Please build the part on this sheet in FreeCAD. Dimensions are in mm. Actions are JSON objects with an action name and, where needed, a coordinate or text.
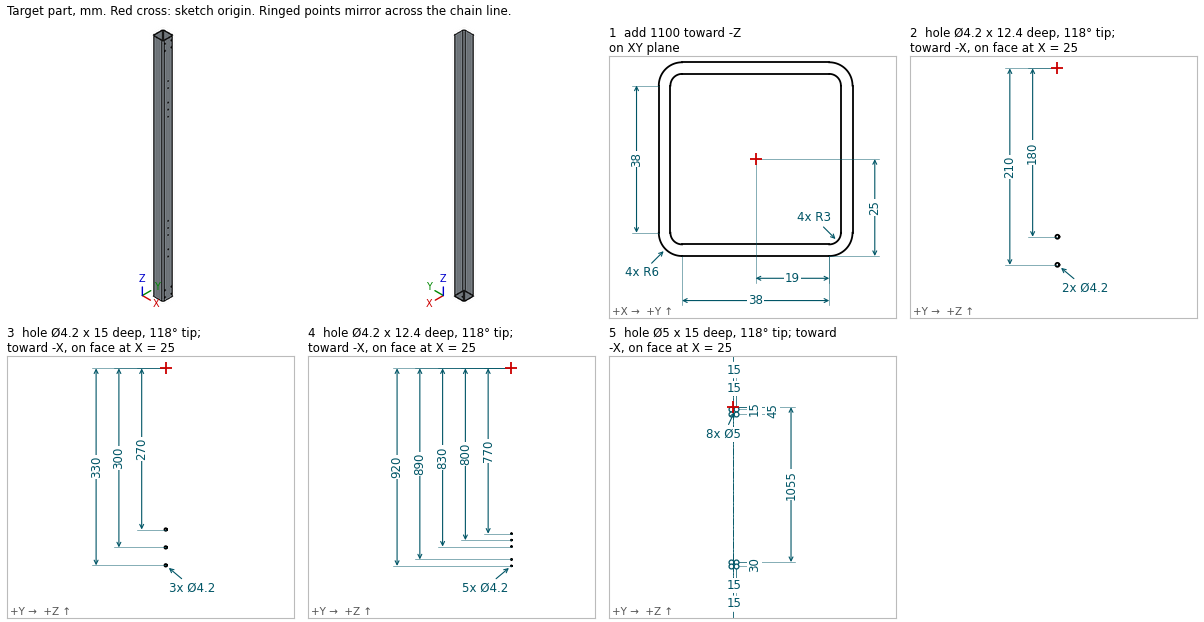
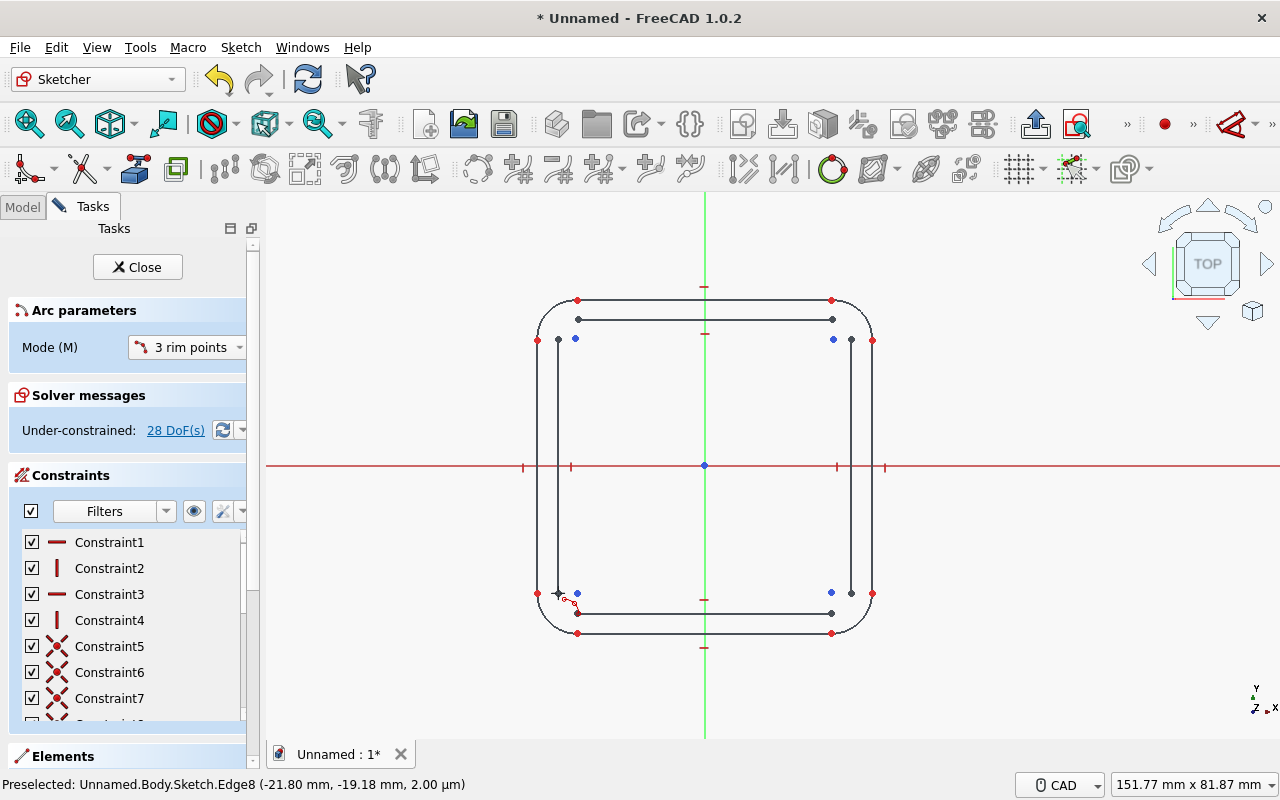
{"action": "left_click", "coordinate": [831, 614]}
{"action": "left_click", "coordinate": [851, 593]}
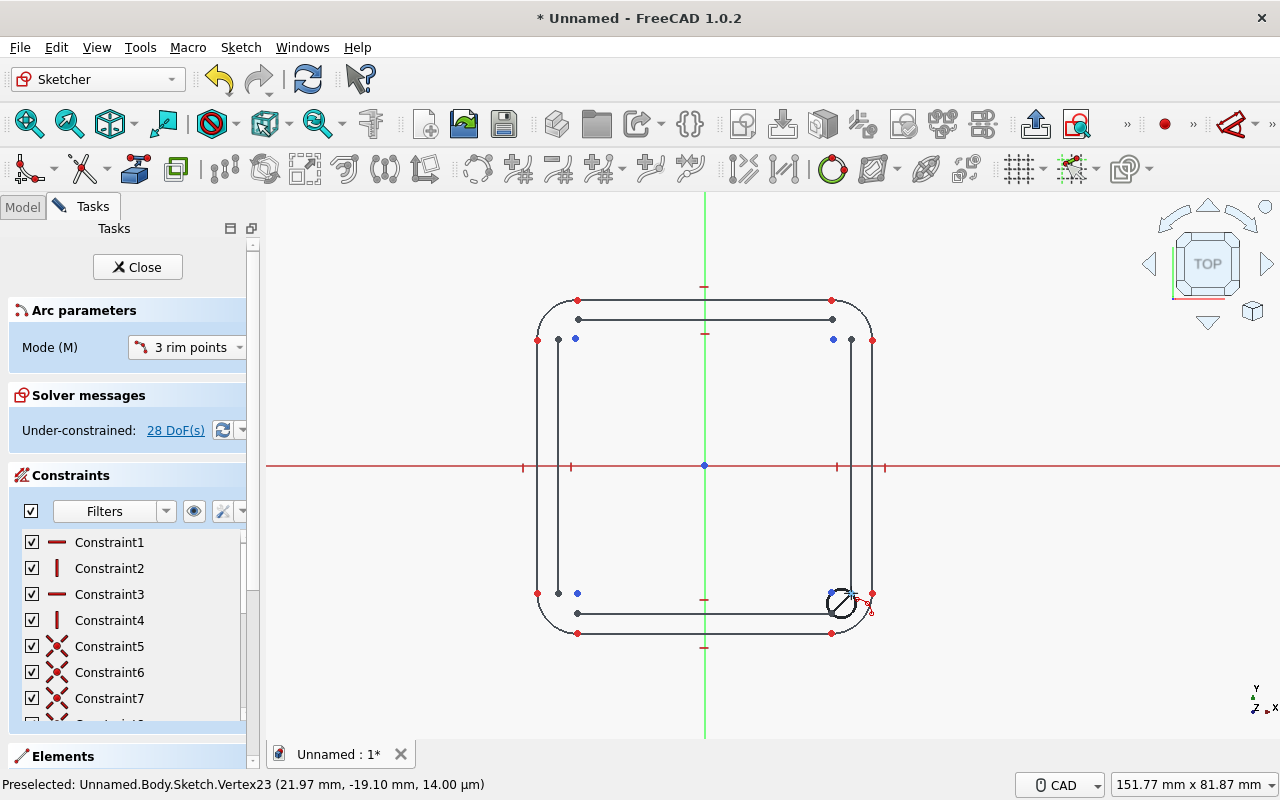
{"action": "scroll", "coordinate": [846, 607], "scroll_direction": "up", "scroll_amount": 5}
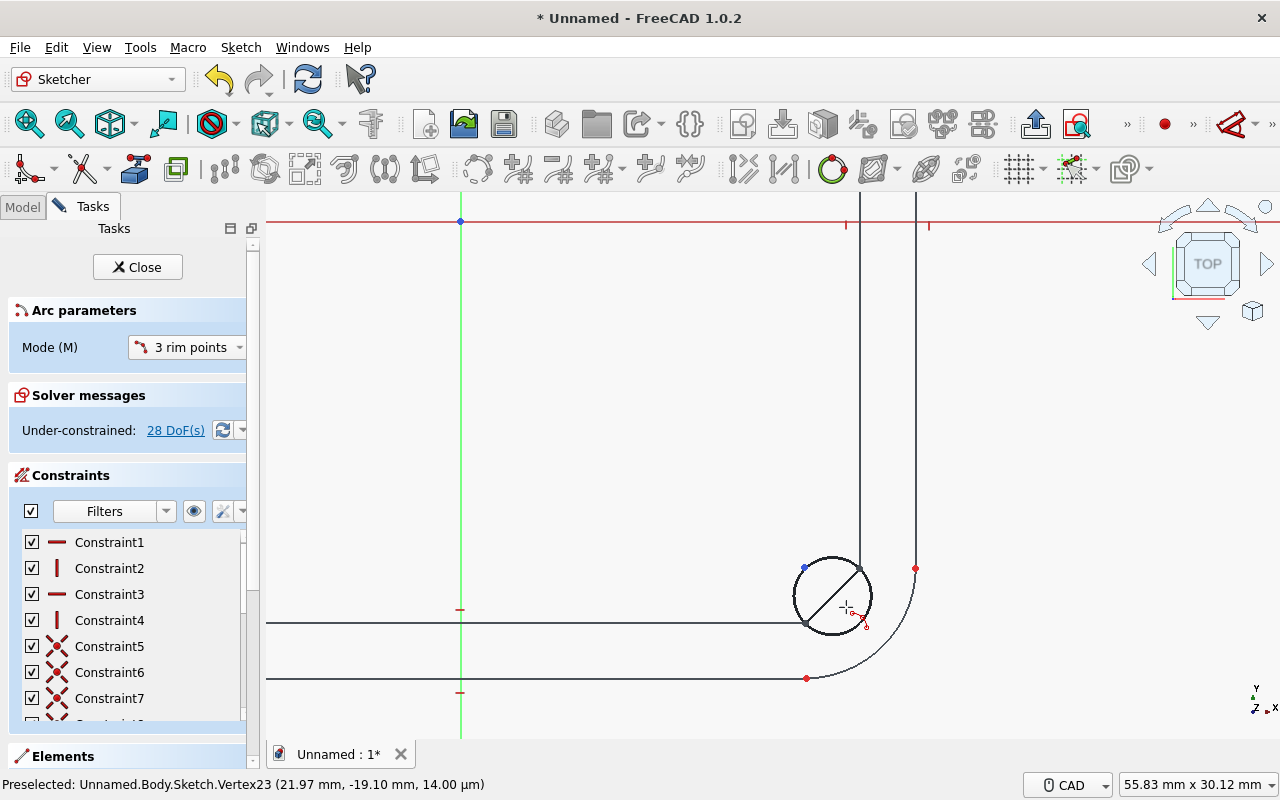
{"action": "left_click", "coordinate": [844, 606]}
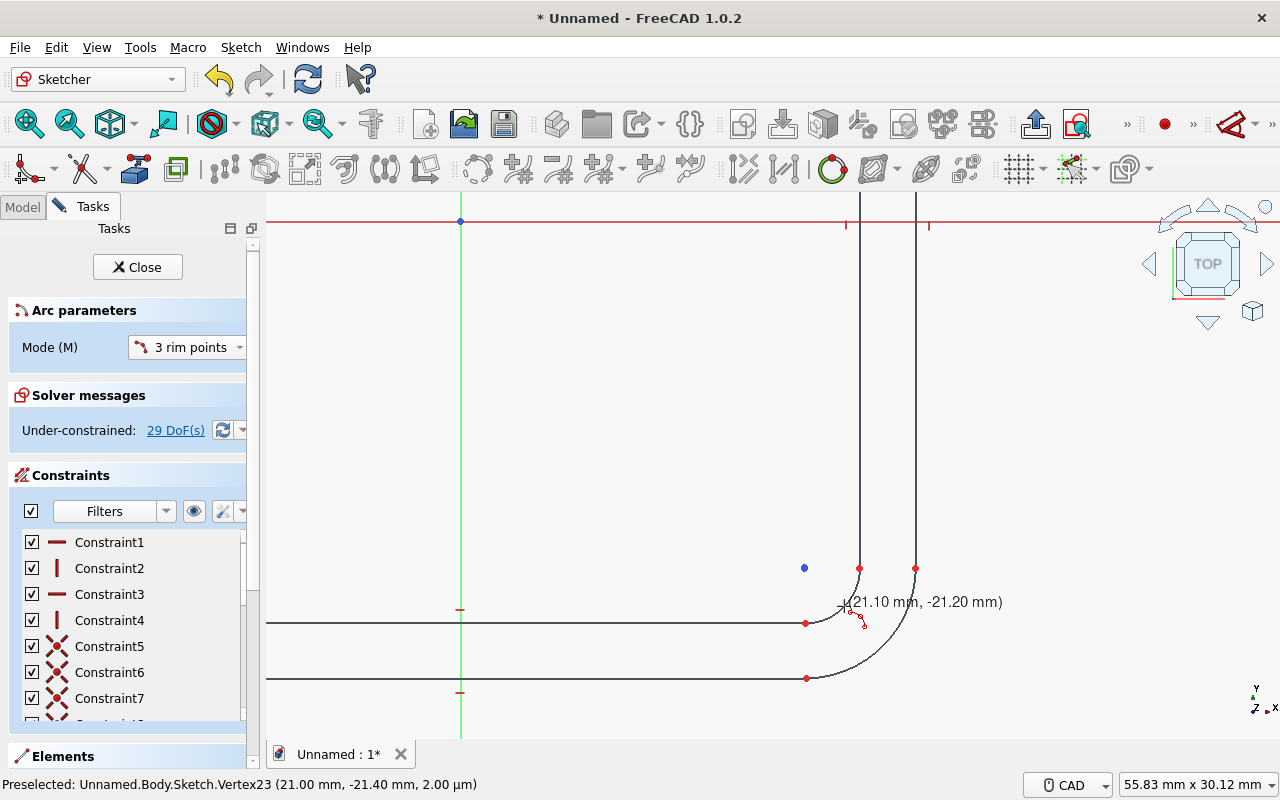
{"action": "scroll", "coordinate": [846, 607], "scroll_direction": "down", "scroll_amount": 5}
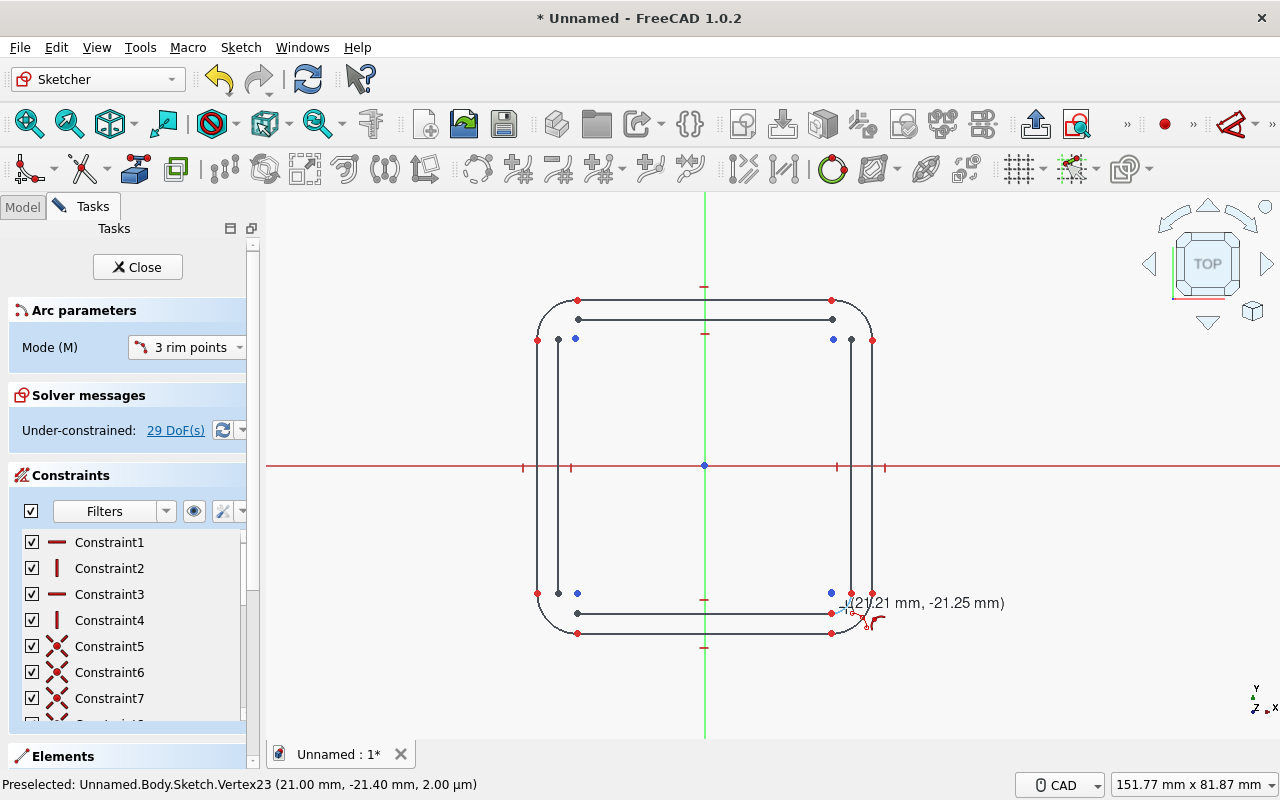
{"action": "left_click", "coordinate": [851, 340]}
{"action": "left_click", "coordinate": [832, 320]}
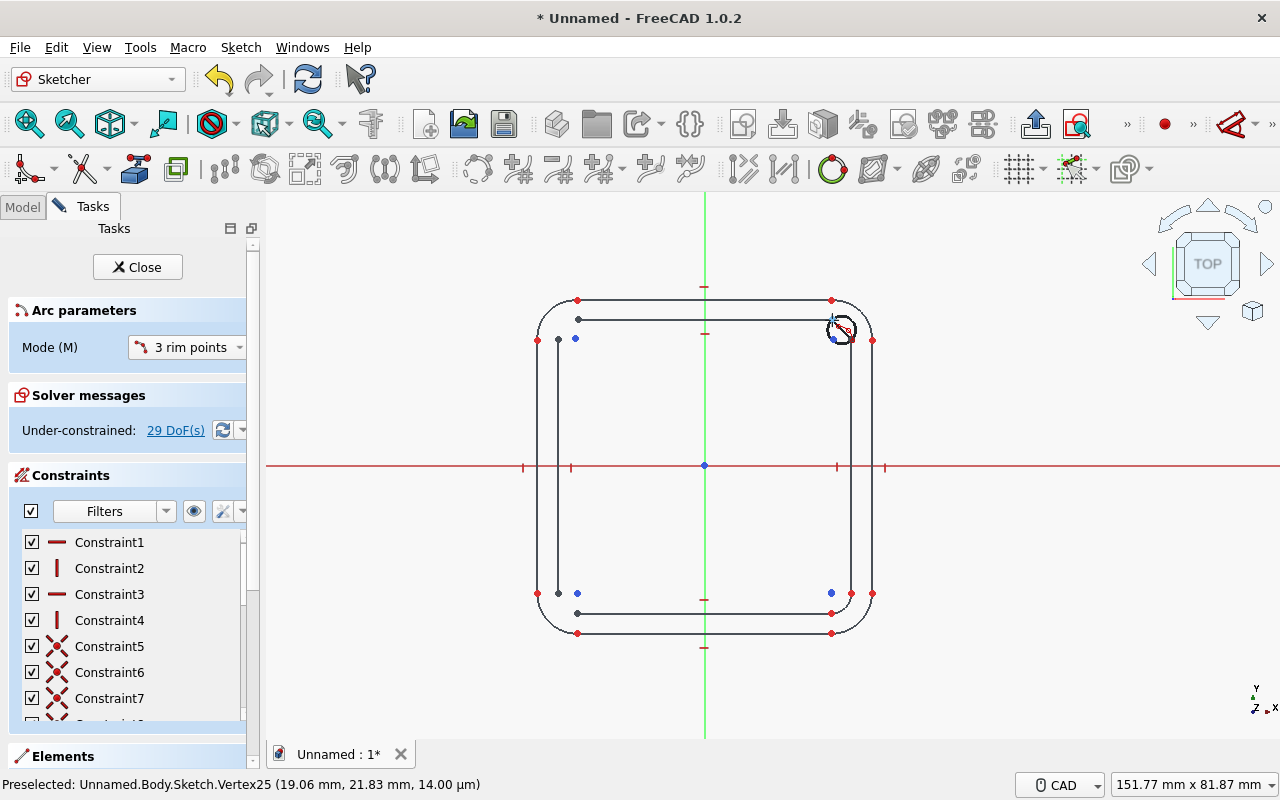
{"action": "scroll", "coordinate": [846, 325], "scroll_direction": "up", "scroll_amount": 5}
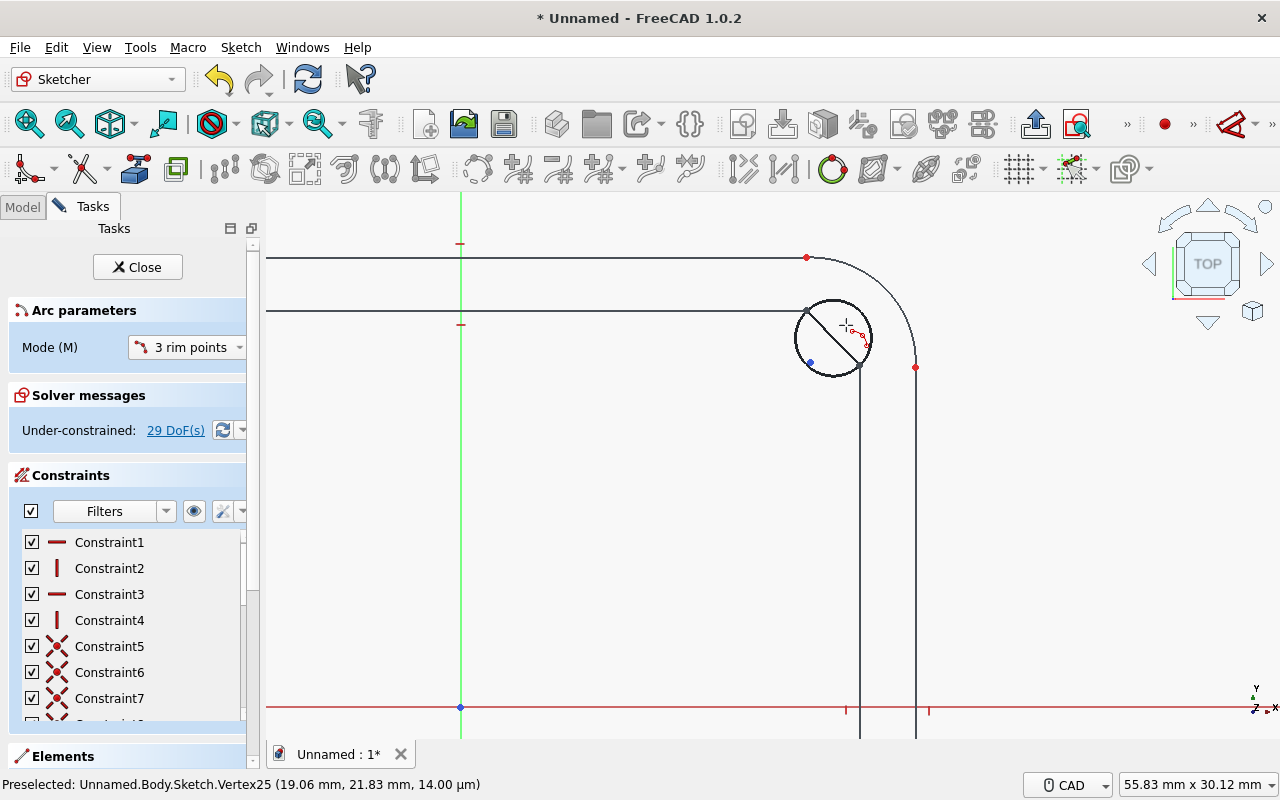
{"action": "left_click", "coordinate": [844, 324]}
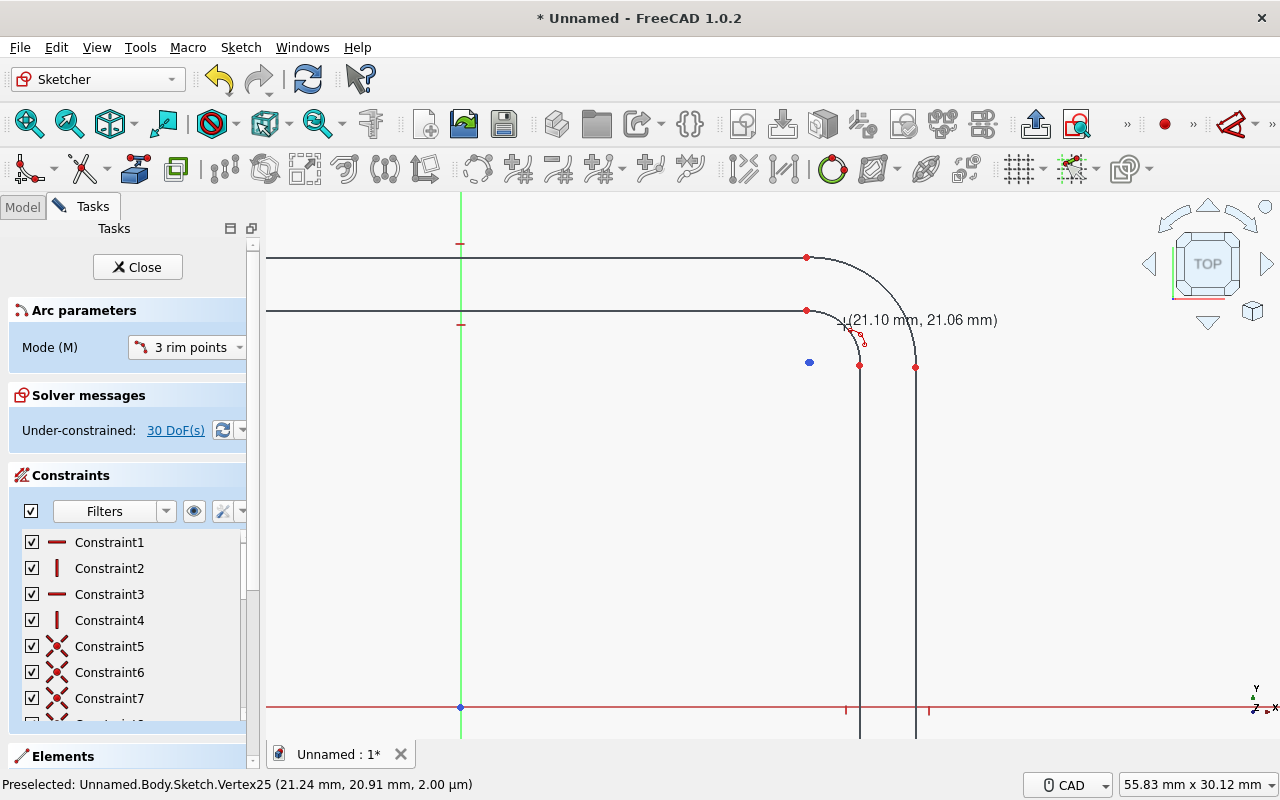
{"action": "scroll", "coordinate": [846, 325], "scroll_direction": "down", "scroll_amount": 5}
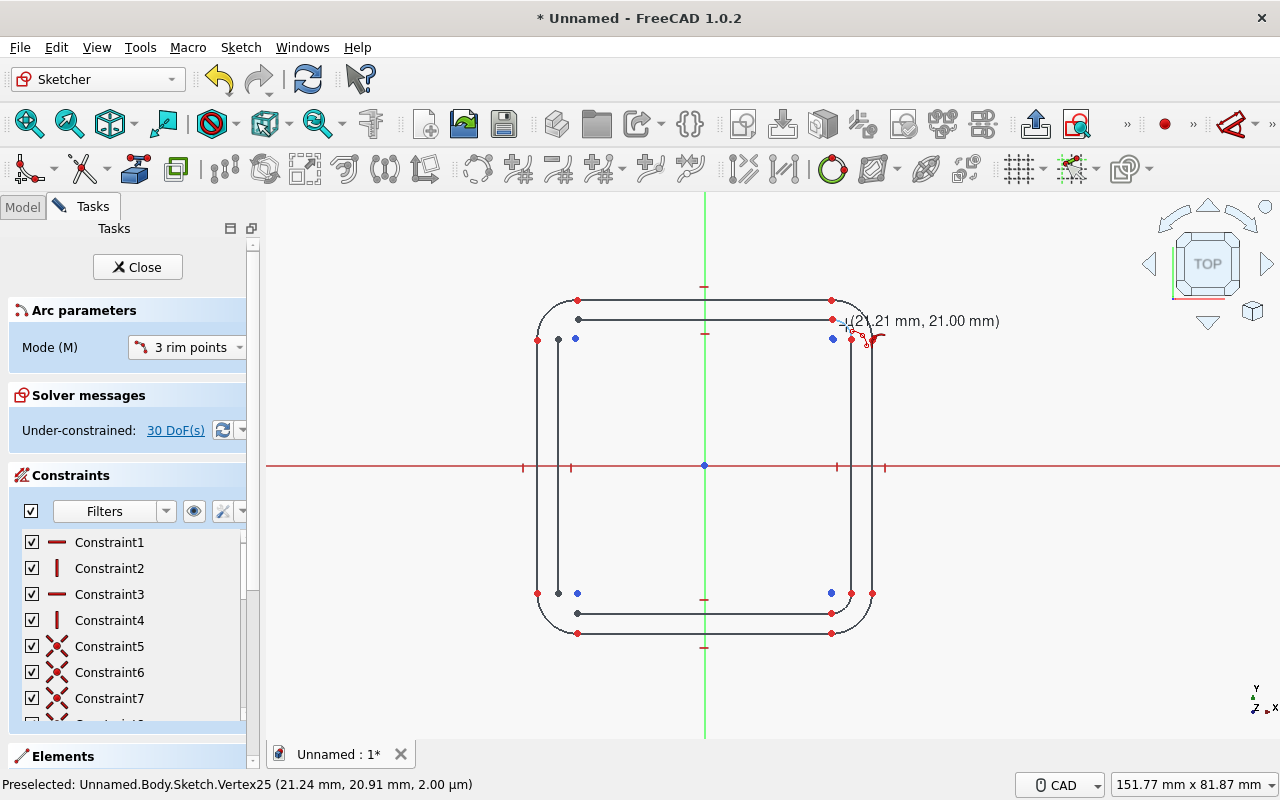
{"action": "left_click", "coordinate": [578, 320]}
{"action": "left_click", "coordinate": [558, 340]}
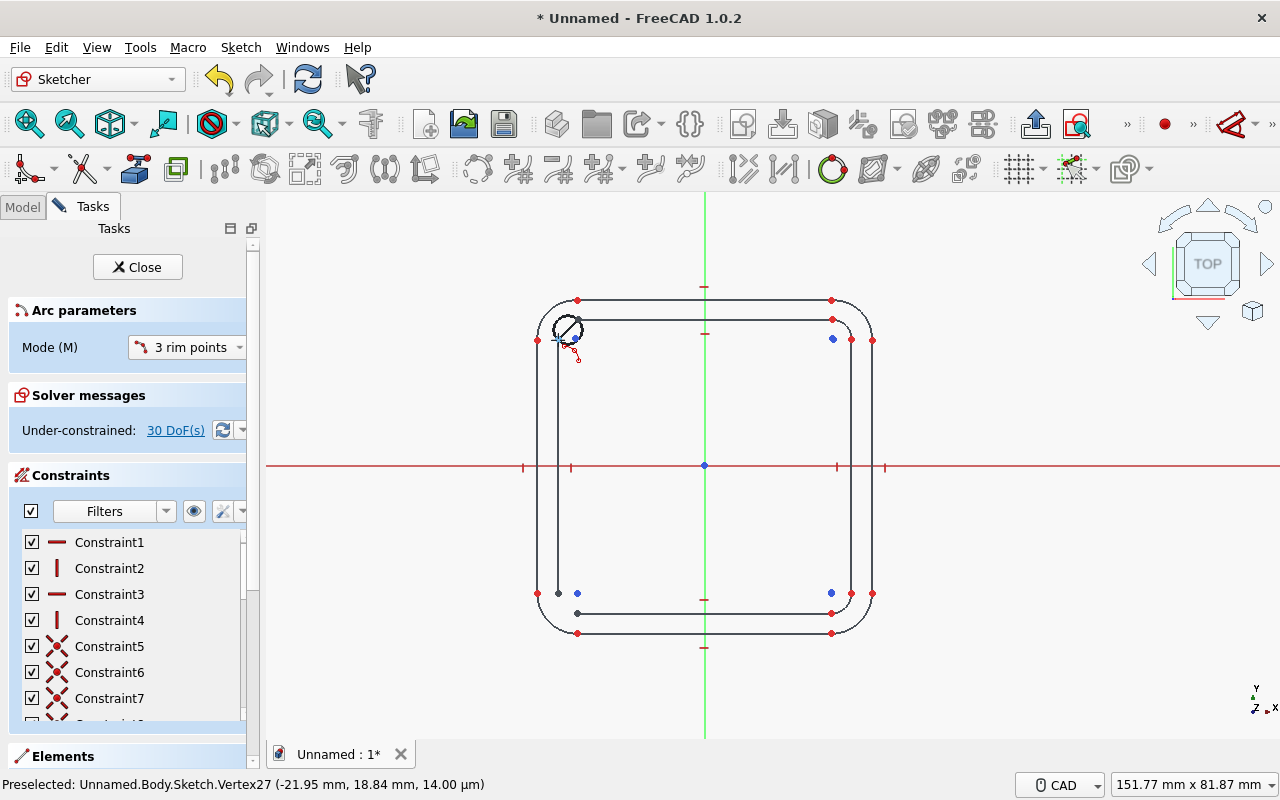
{"action": "scroll", "coordinate": [564, 325], "scroll_direction": "up", "scroll_amount": 5}